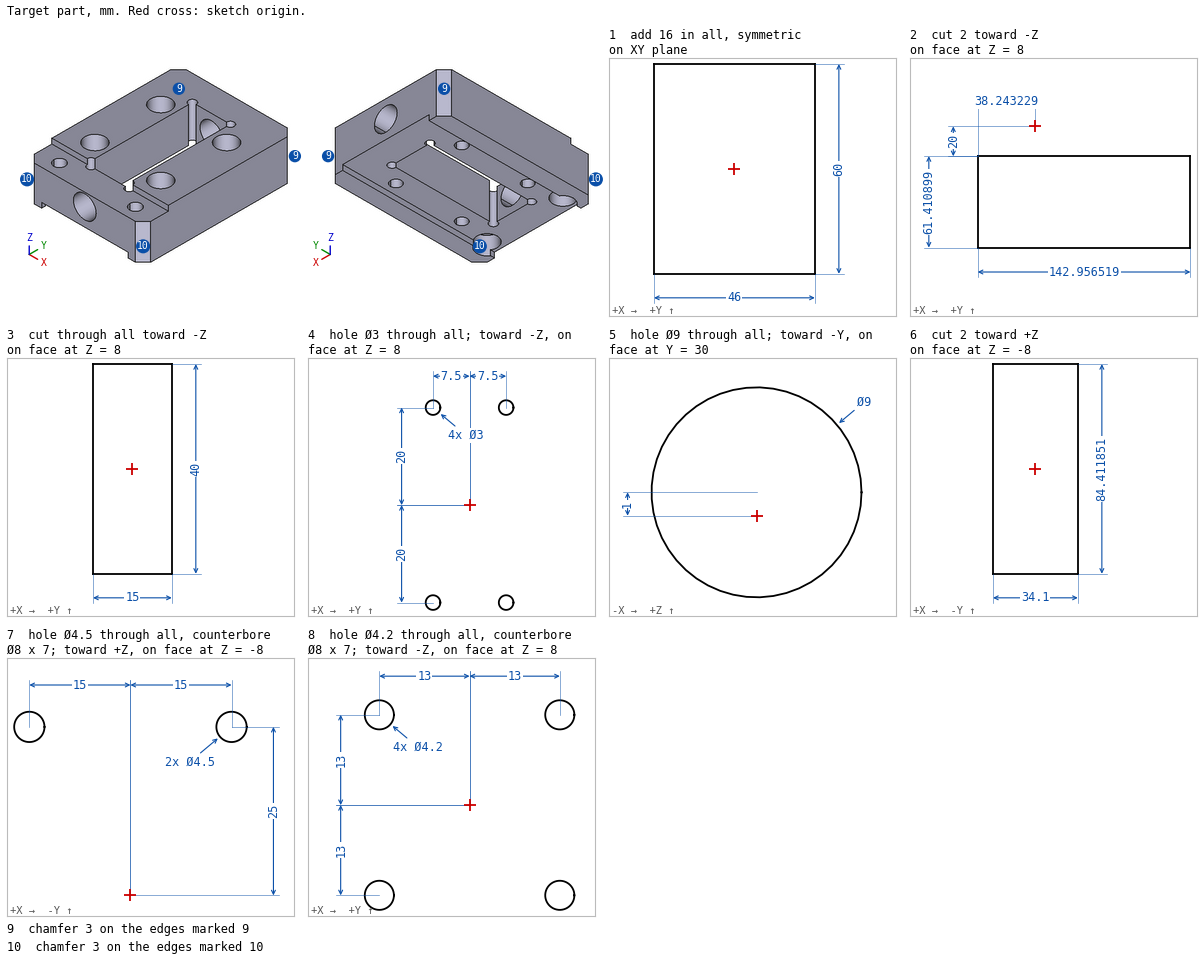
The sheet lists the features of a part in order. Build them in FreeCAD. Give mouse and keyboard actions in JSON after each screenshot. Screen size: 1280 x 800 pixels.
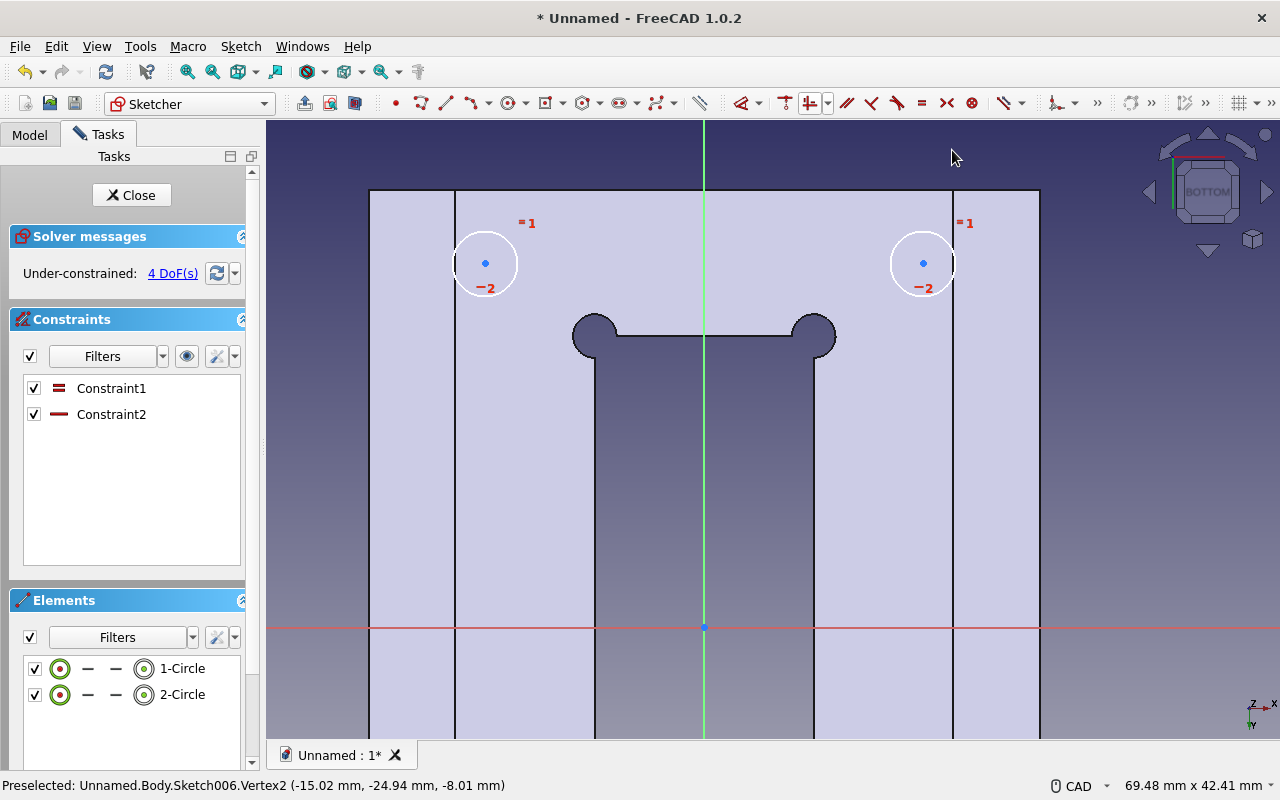
{"action": "left_click", "coordinate": [740, 104]}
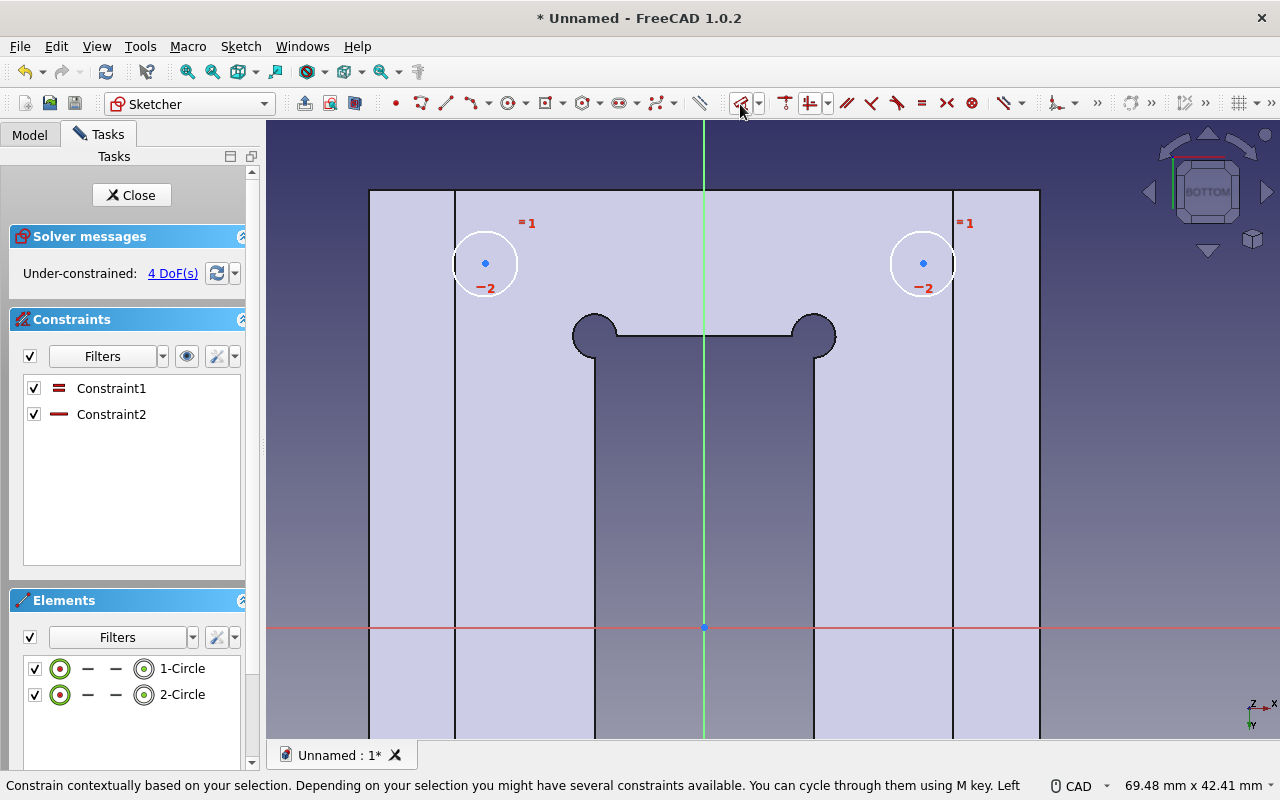
{"action": "left_click", "coordinate": [946, 241]}
{"action": "left_click", "coordinate": [969, 218]}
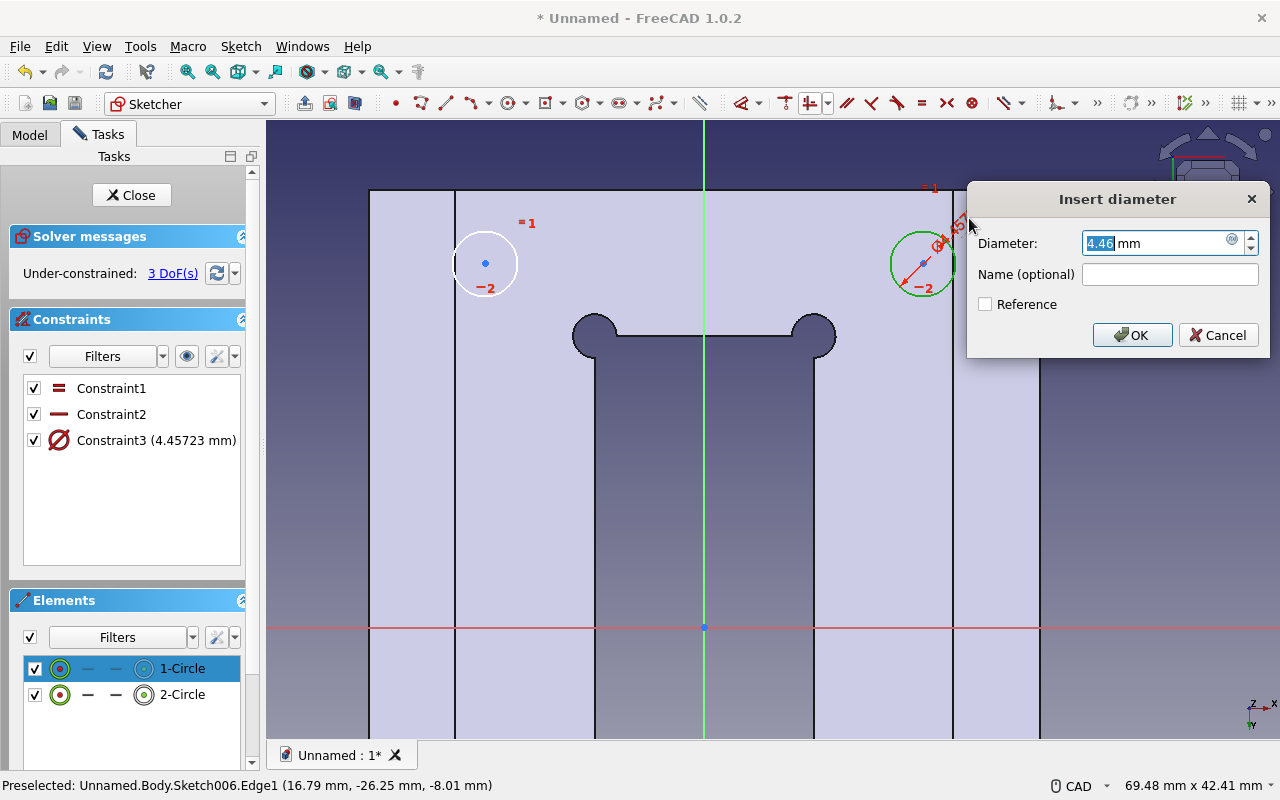
{"action": "type", "text": "4.5"}
{"action": "key", "text": "Return"}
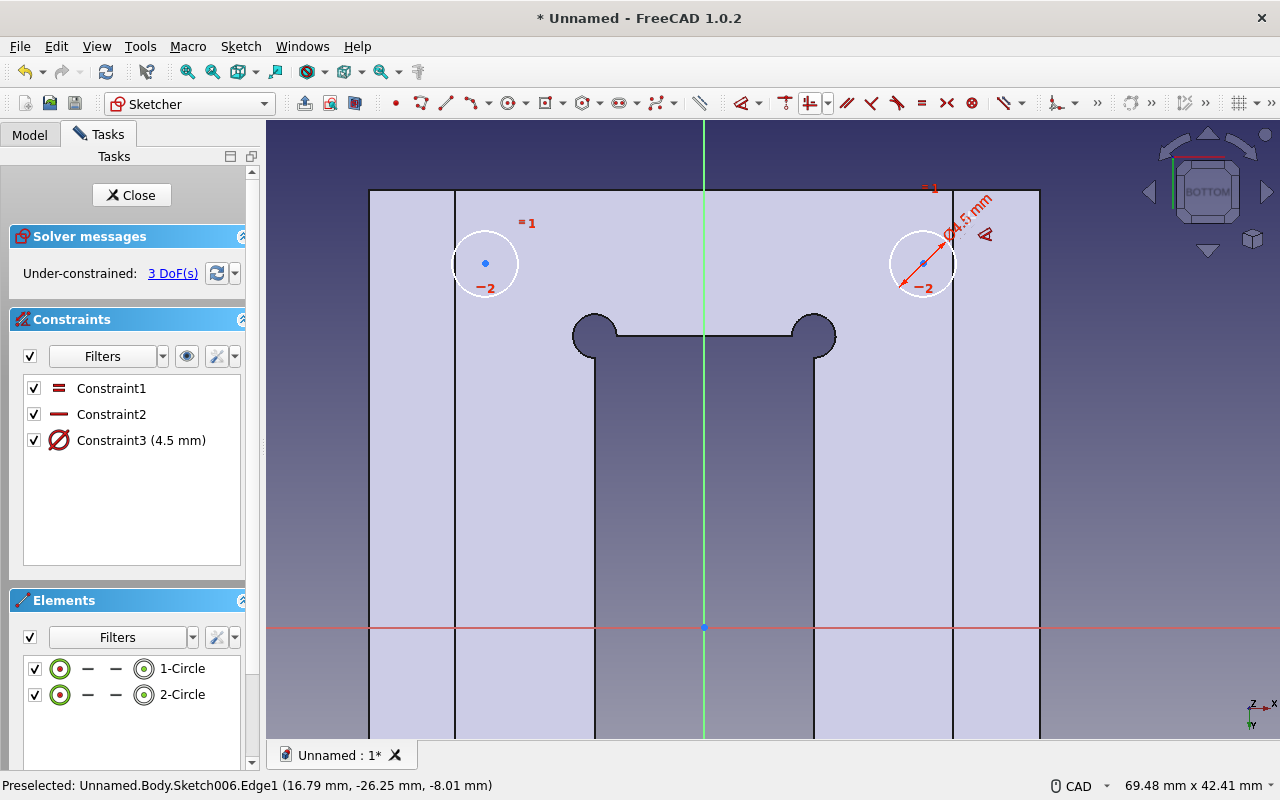
{"action": "left_click", "coordinate": [923, 264]}
{"action": "left_click", "coordinate": [814, 662]}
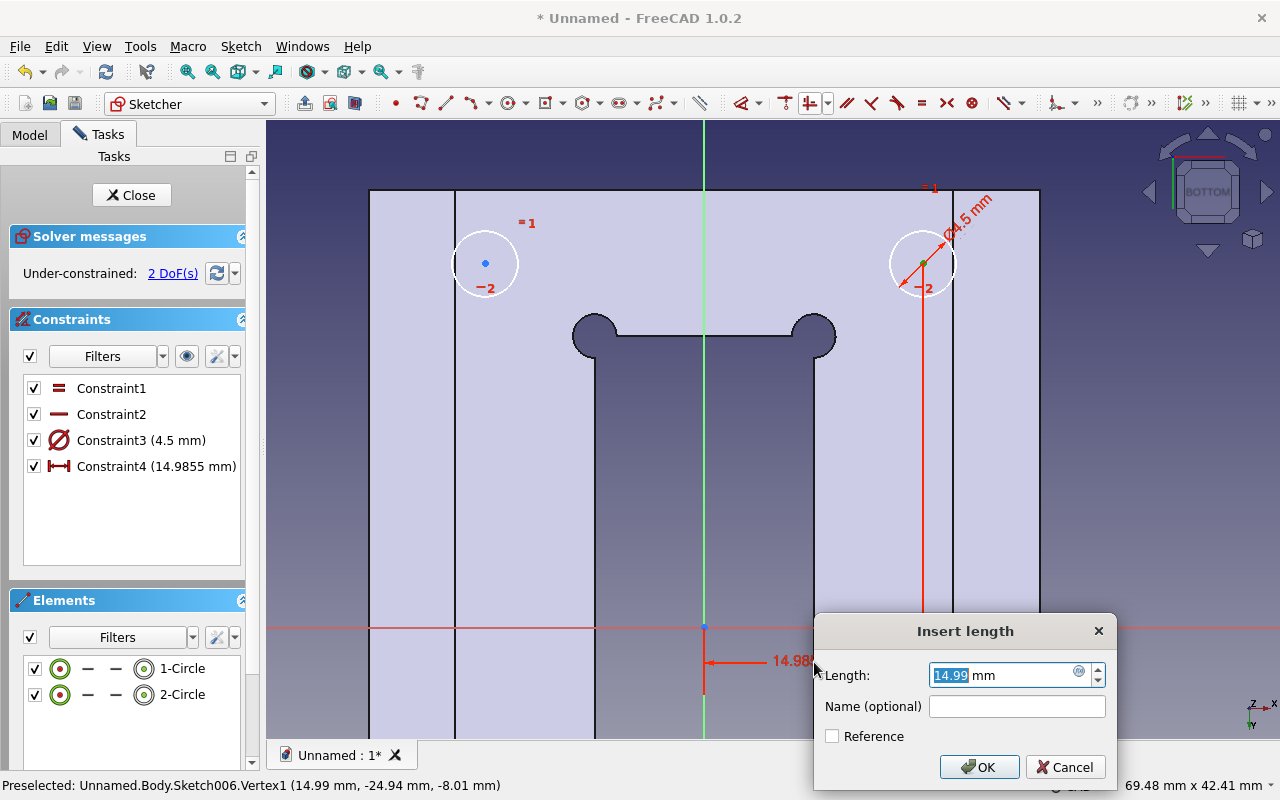
{"action": "type", "text": "15"}
{"action": "key", "text": "Return"}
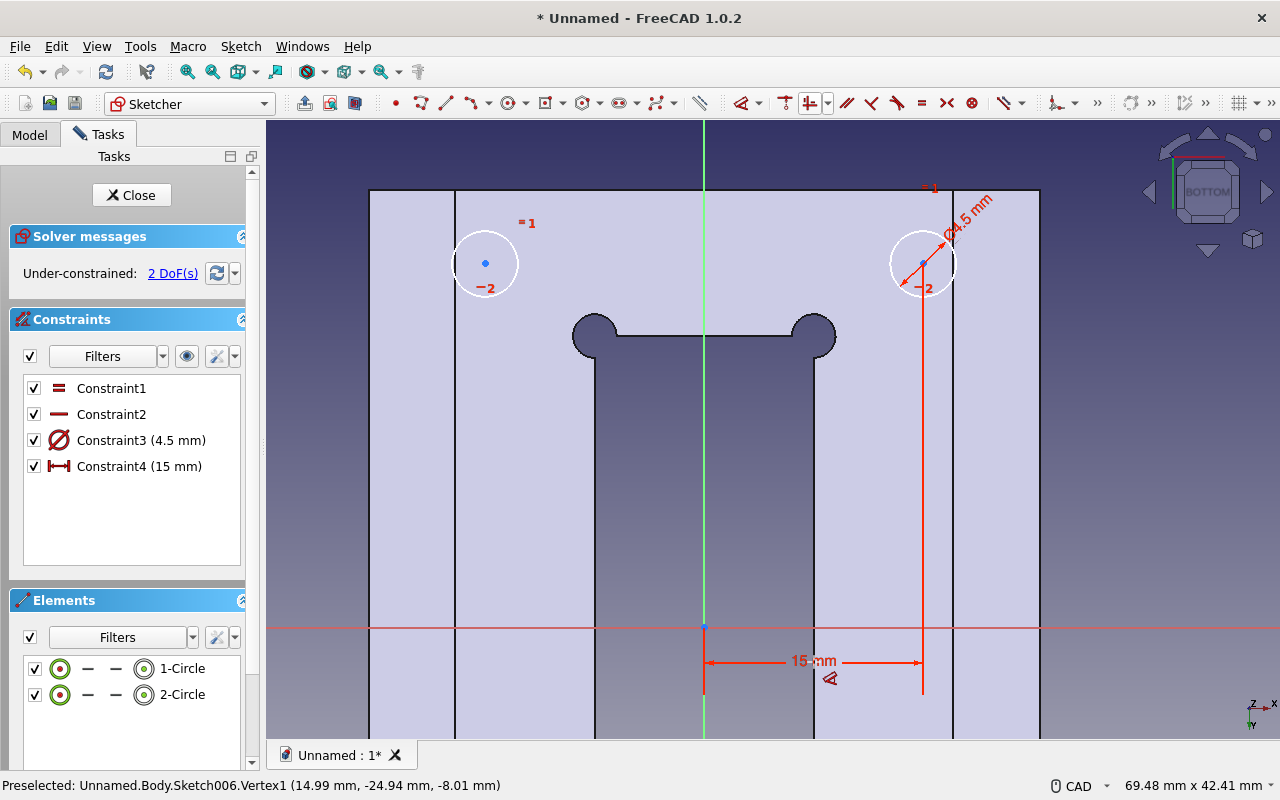
{"action": "left_click", "coordinate": [923, 264]}
{"action": "left_click", "coordinate": [957, 446]}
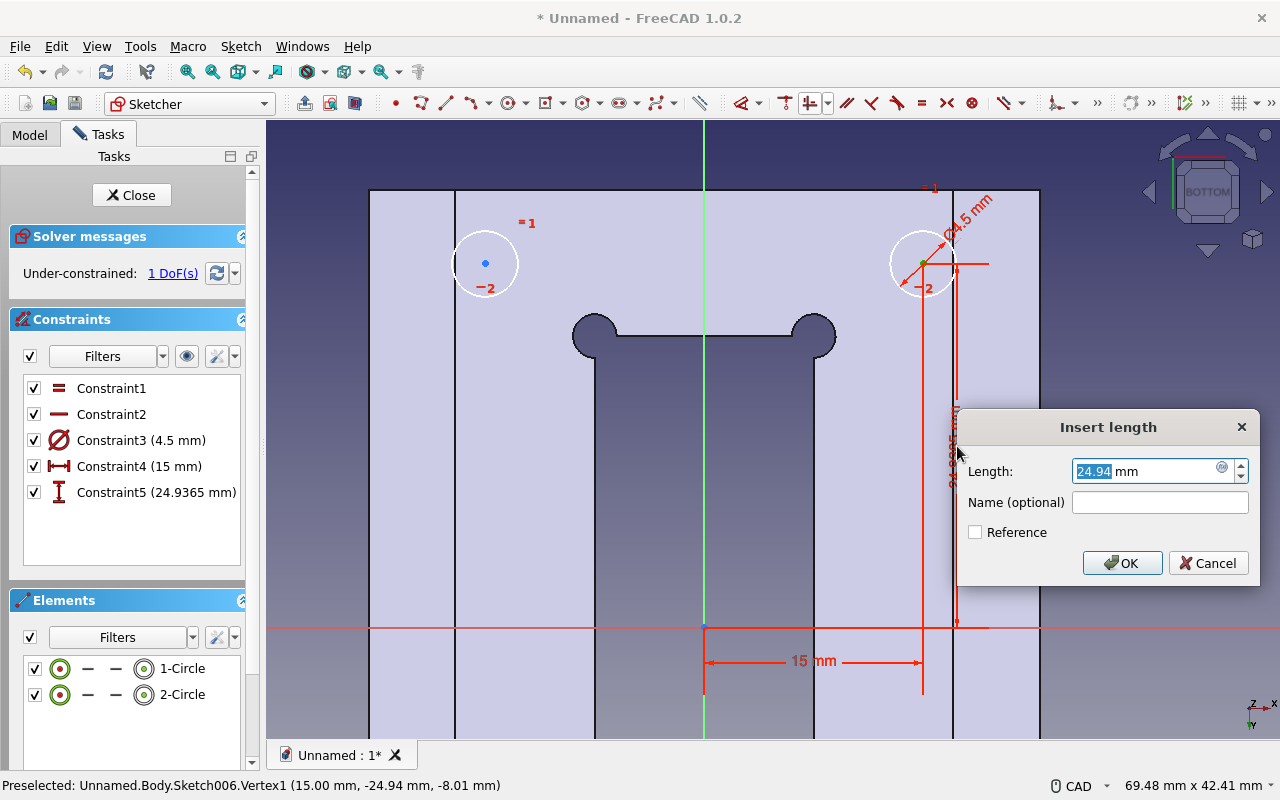
{"action": "type", "text": "25"}
{"action": "key", "text": "Return"}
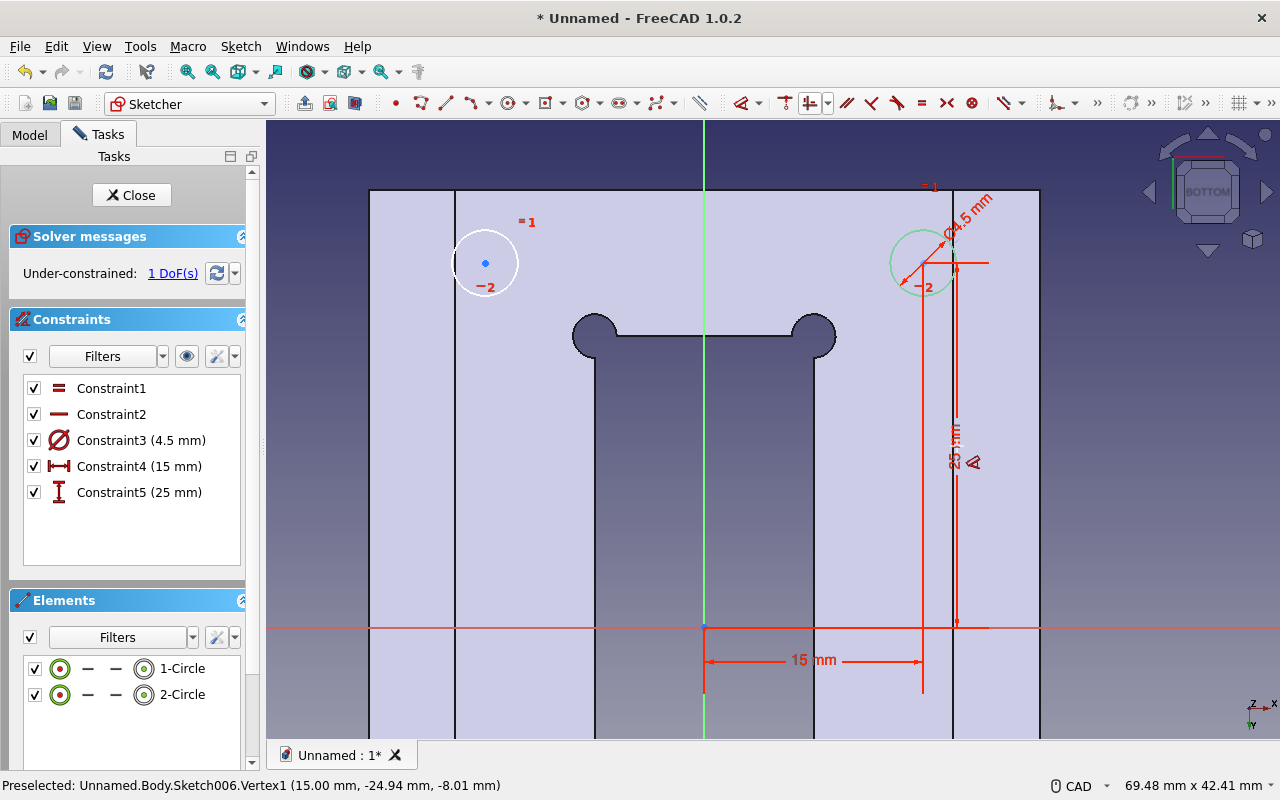
{"action": "left_click", "coordinate": [485, 263]}
{"action": "left_click", "coordinate": [595, 662]}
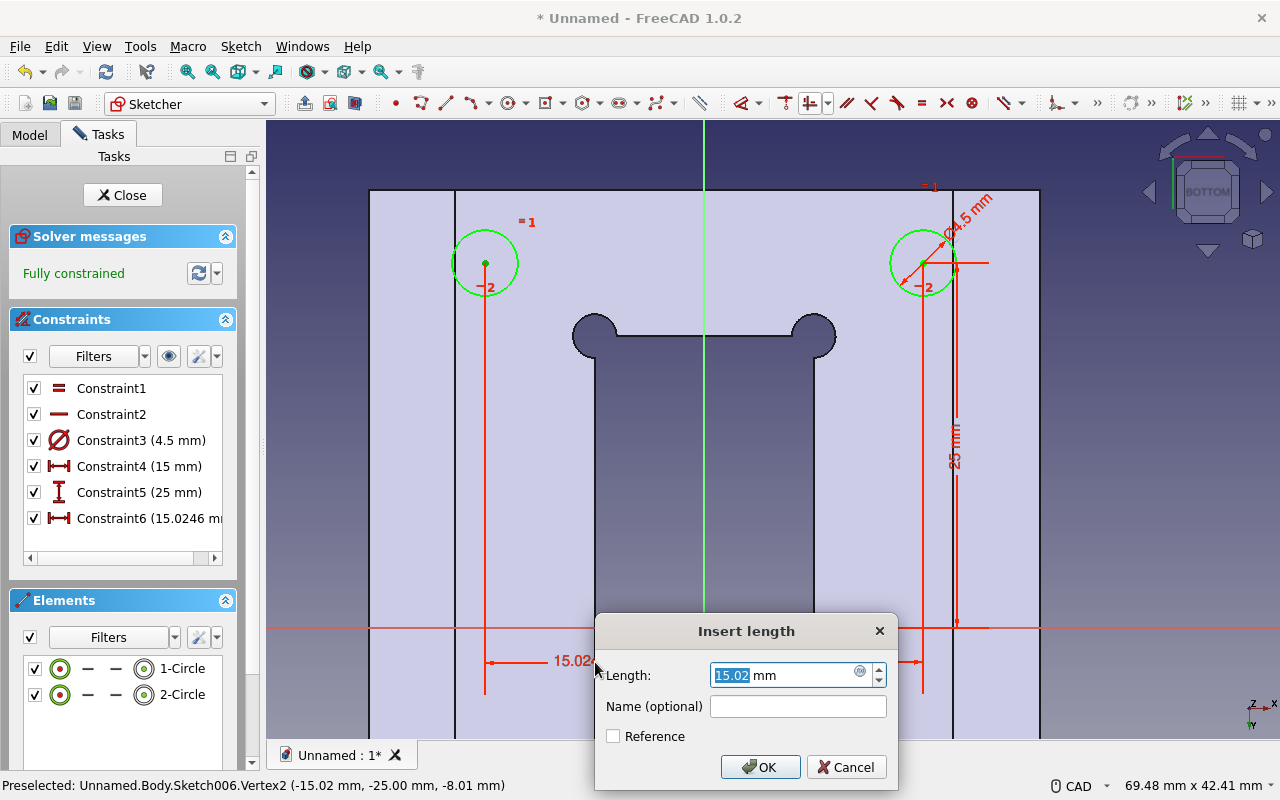
{"action": "type", "text": "15"}
{"action": "key", "text": "Return"}
{"action": "key", "text": "Escape"}